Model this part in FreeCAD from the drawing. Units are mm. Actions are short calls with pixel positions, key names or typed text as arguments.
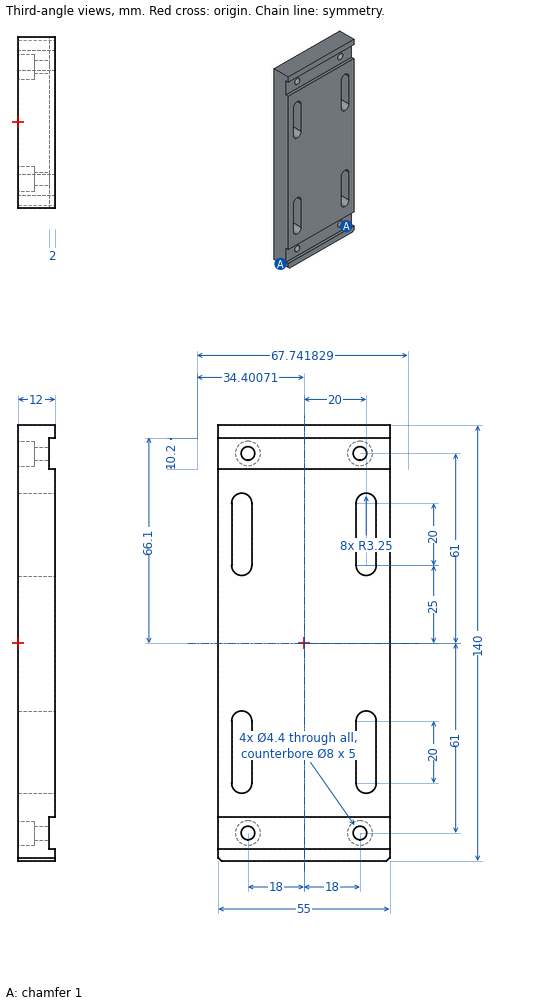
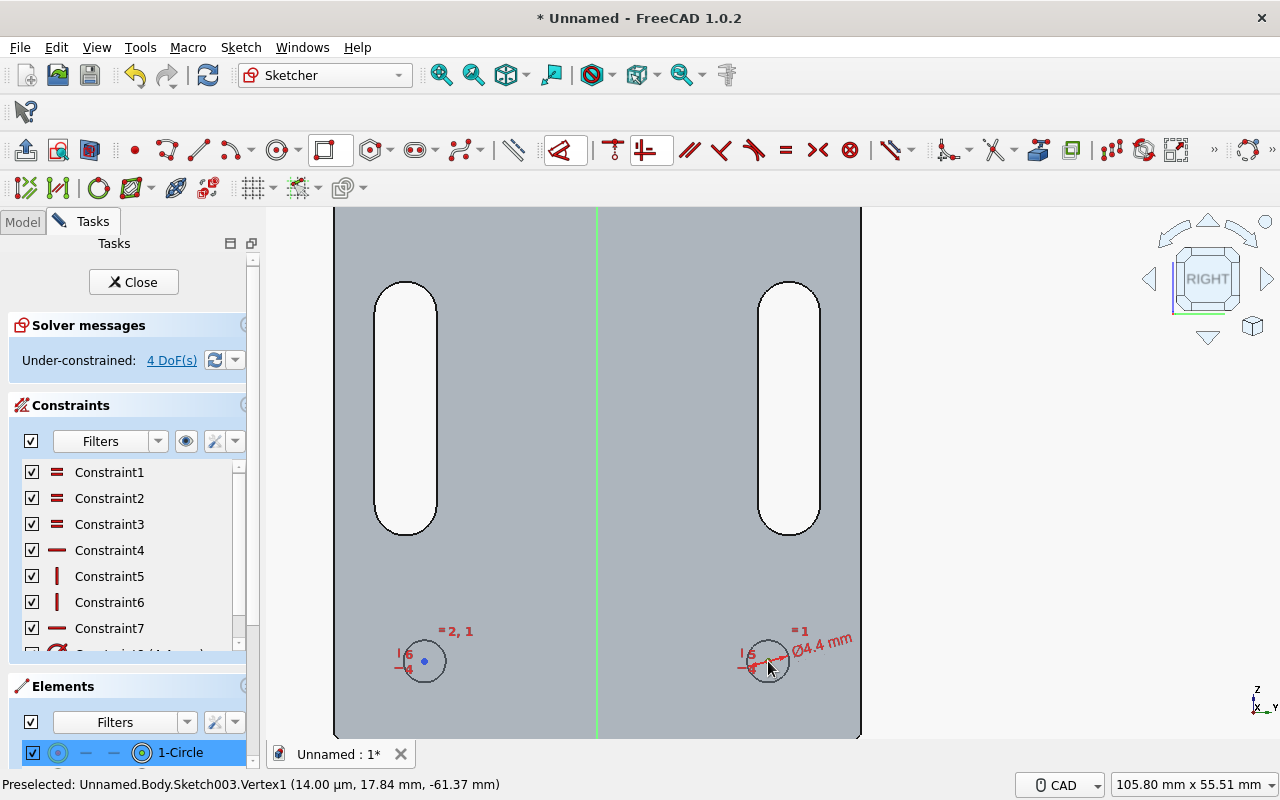
key(l)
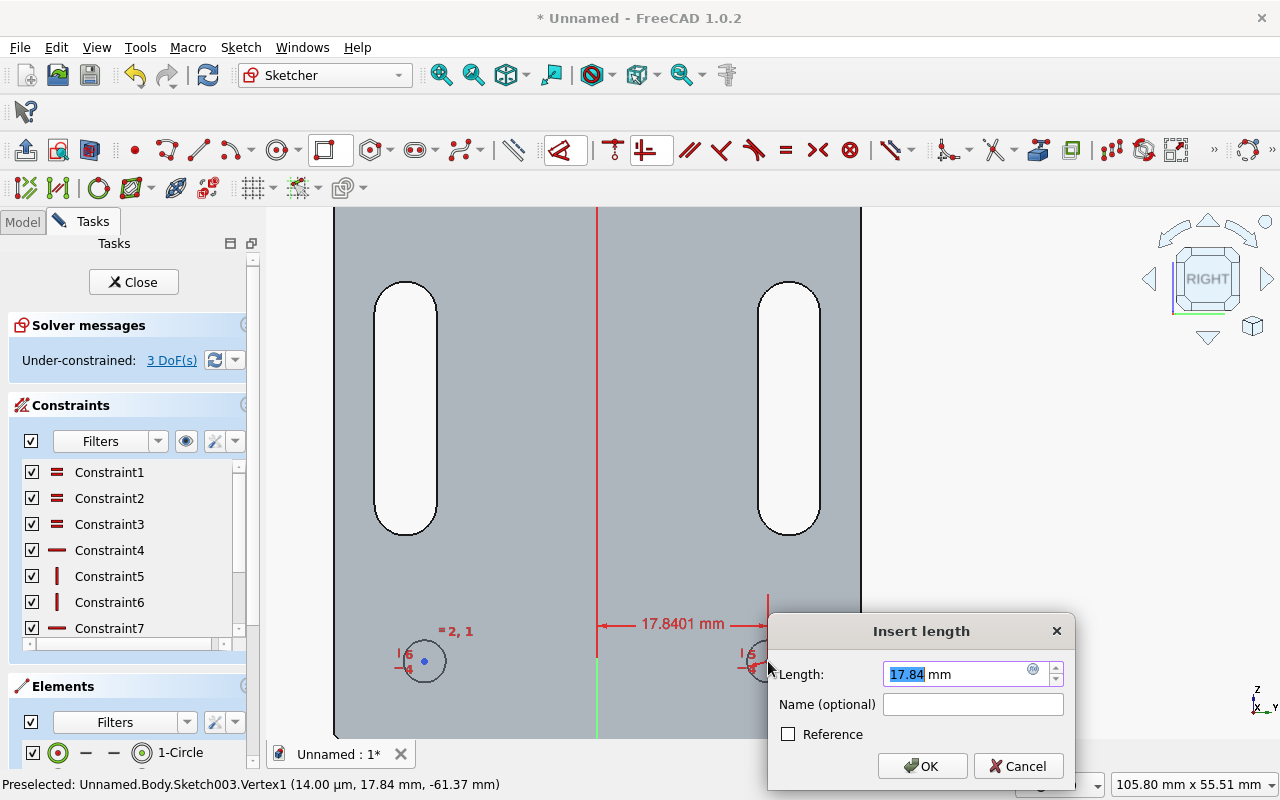
text(18)
key(Return)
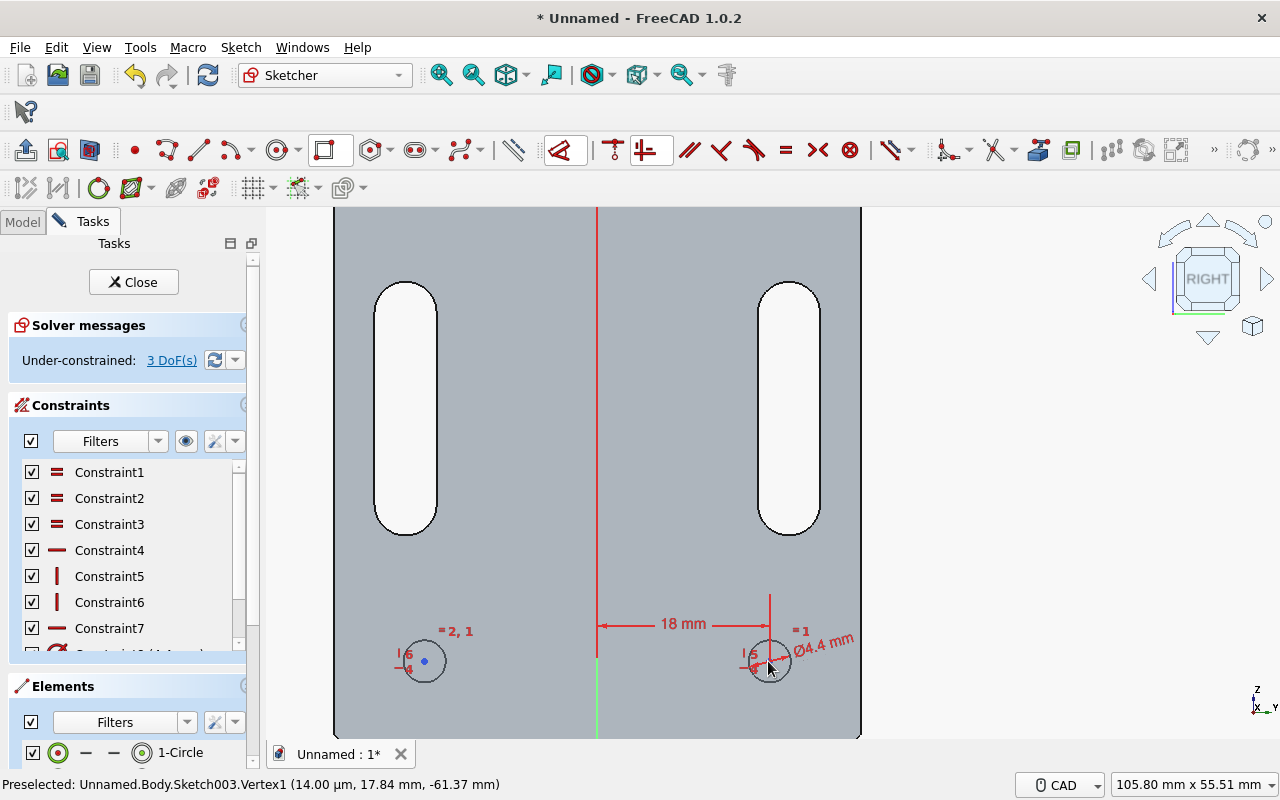
click(770, 661)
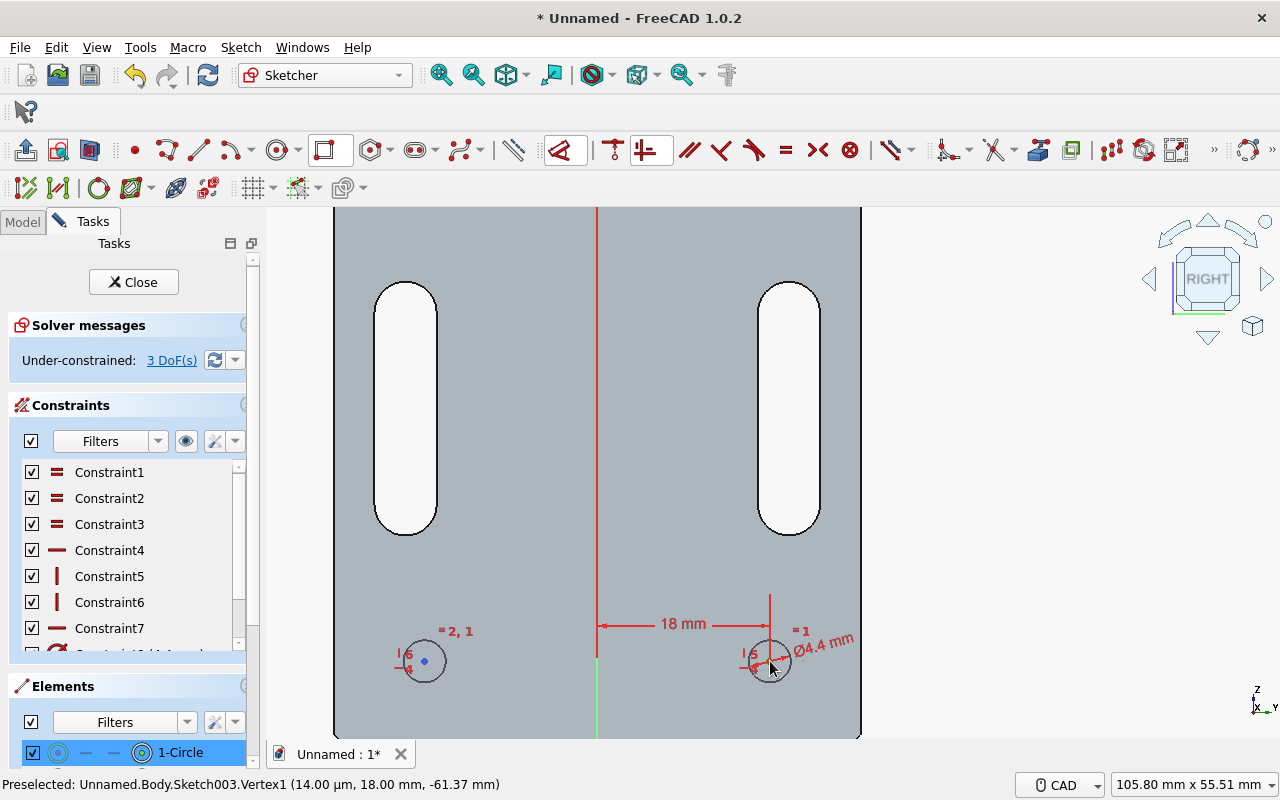
key(i)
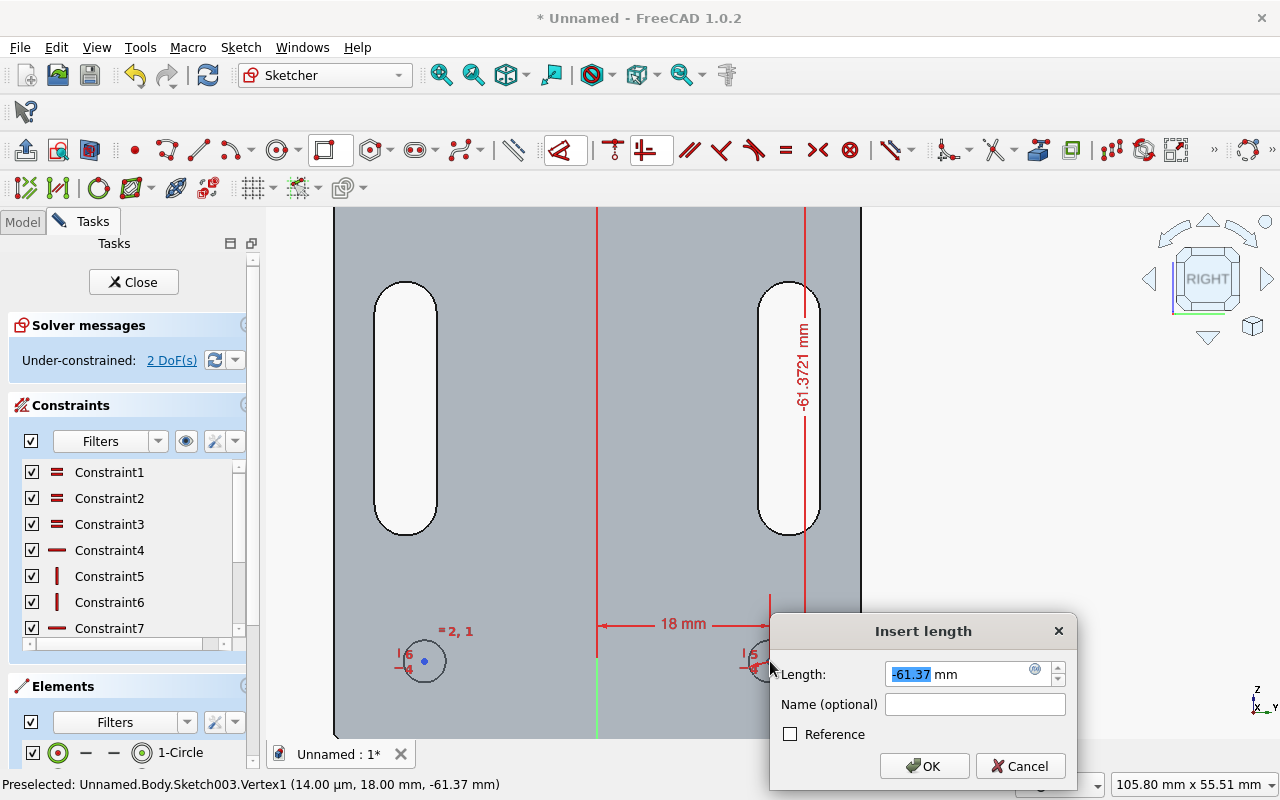
text(-61)
key(Return)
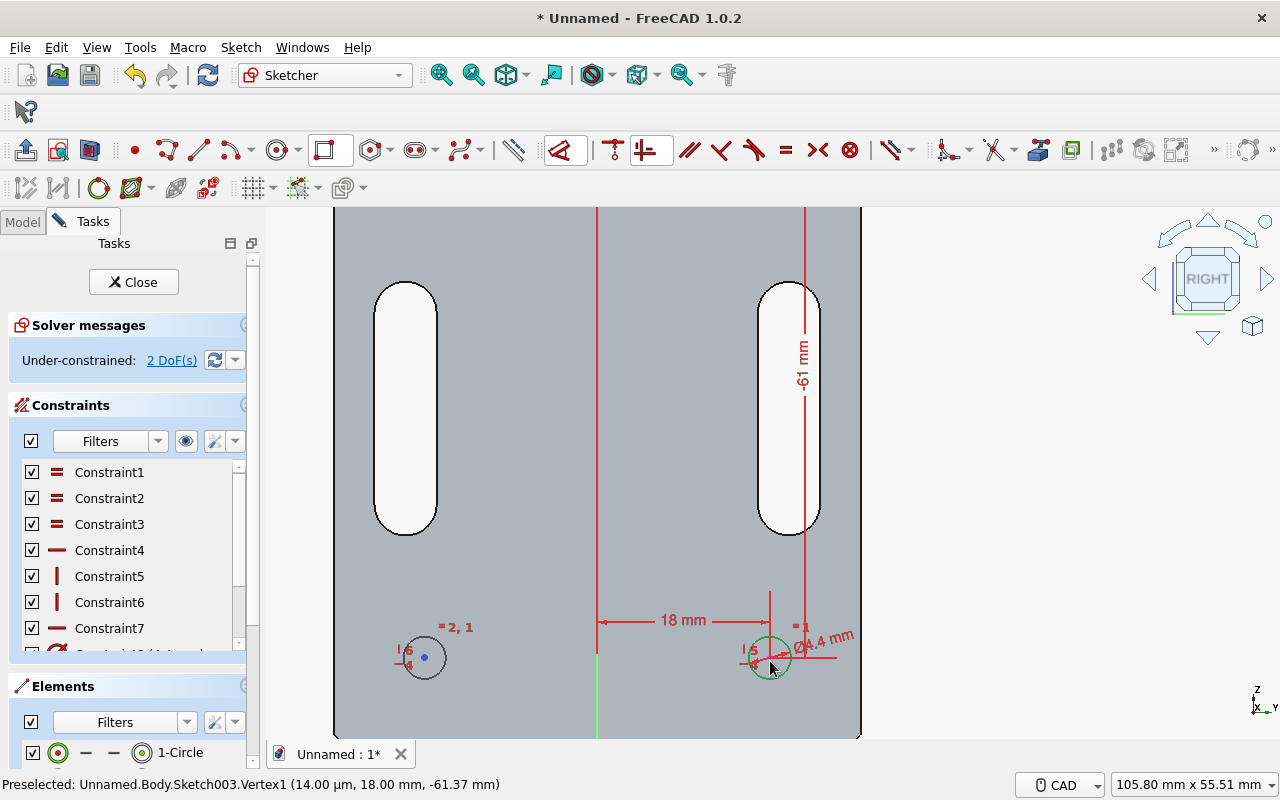
click(425, 658)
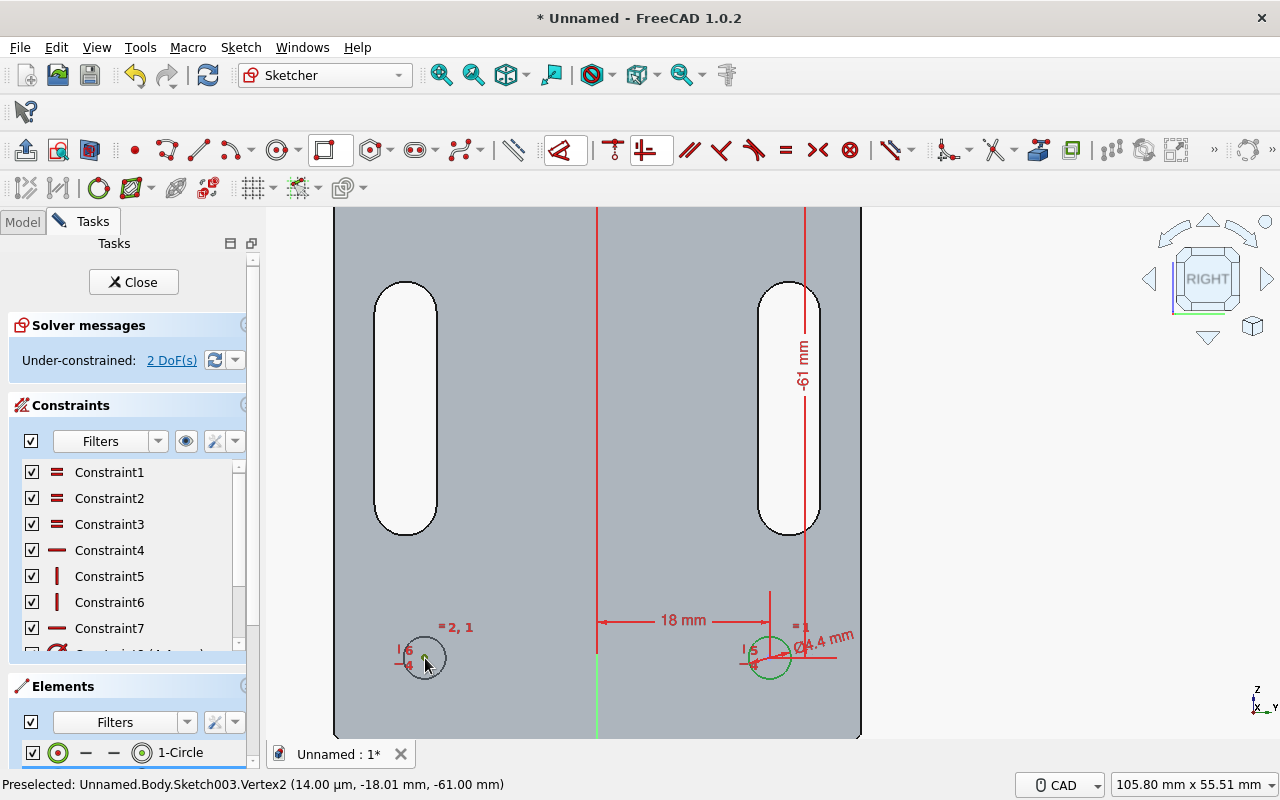
click(582, 150)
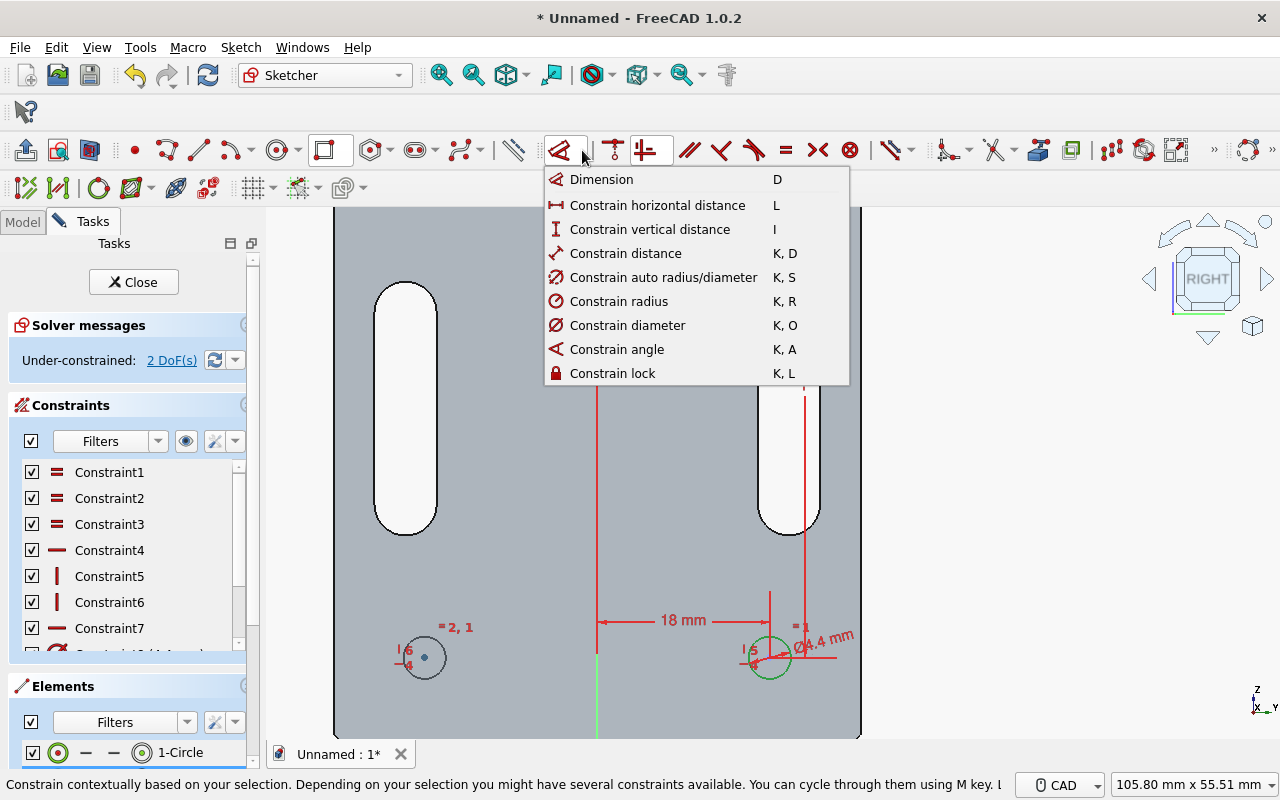
click(697, 205)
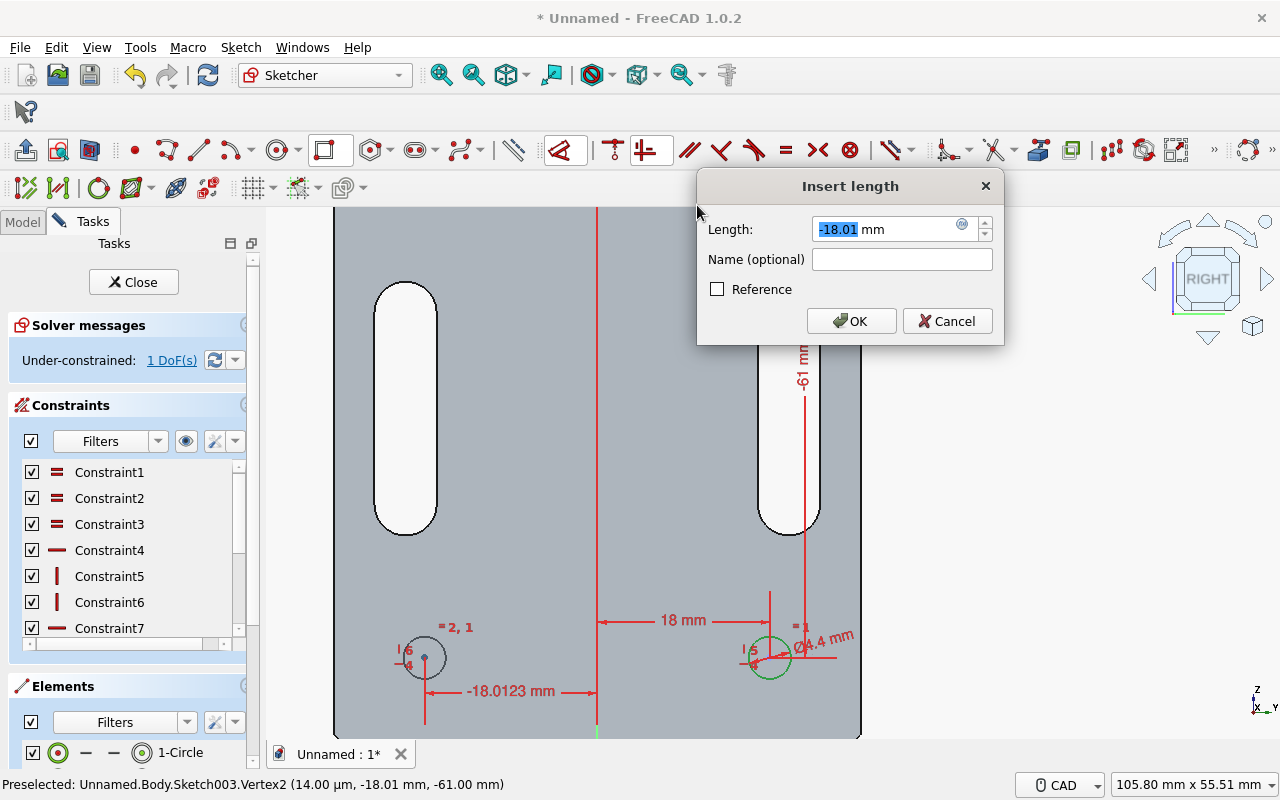
text(-18)
key(Return)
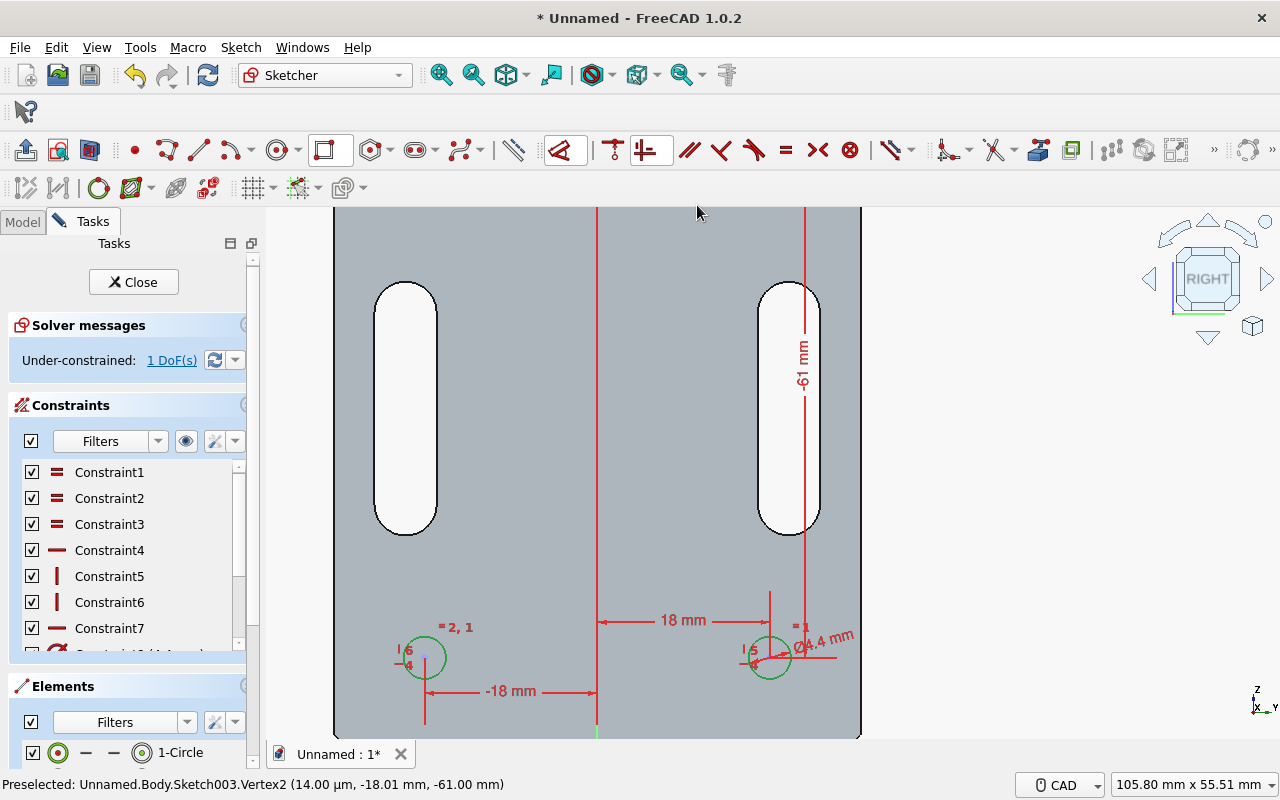
scroll(751, 645, down, 6)